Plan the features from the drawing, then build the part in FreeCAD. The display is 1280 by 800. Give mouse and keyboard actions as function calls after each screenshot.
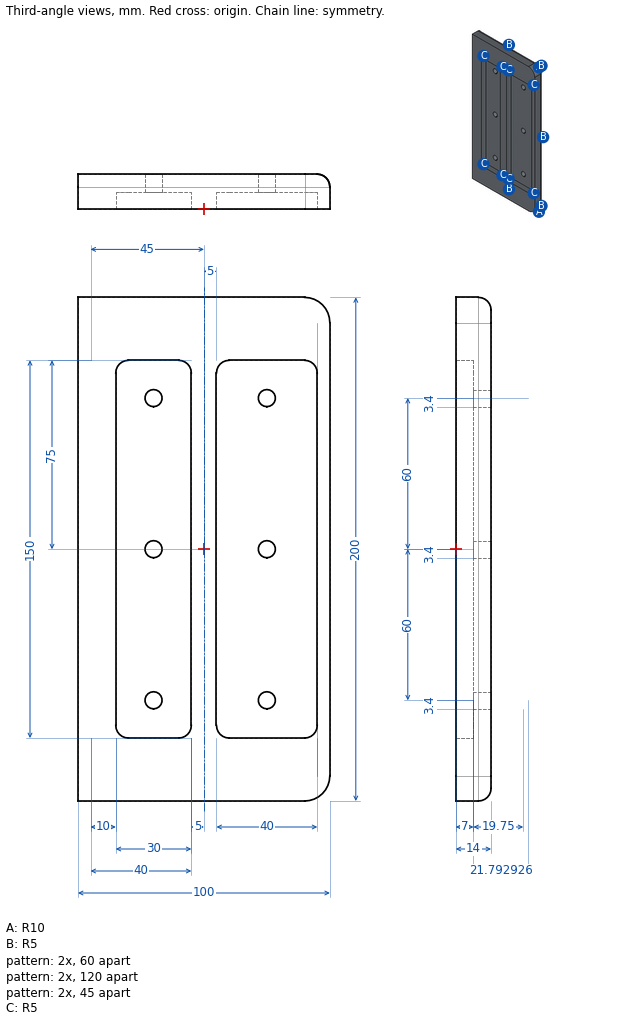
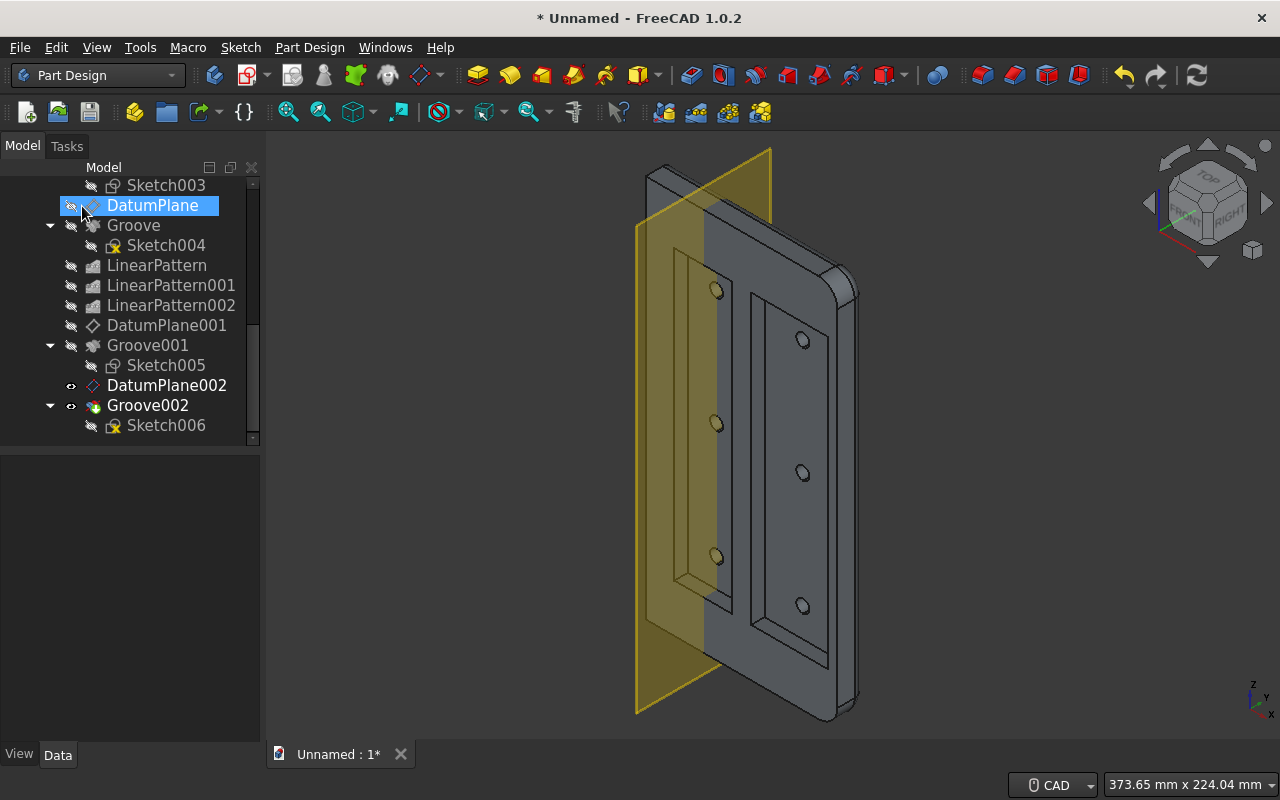
click(116, 386)
key(space)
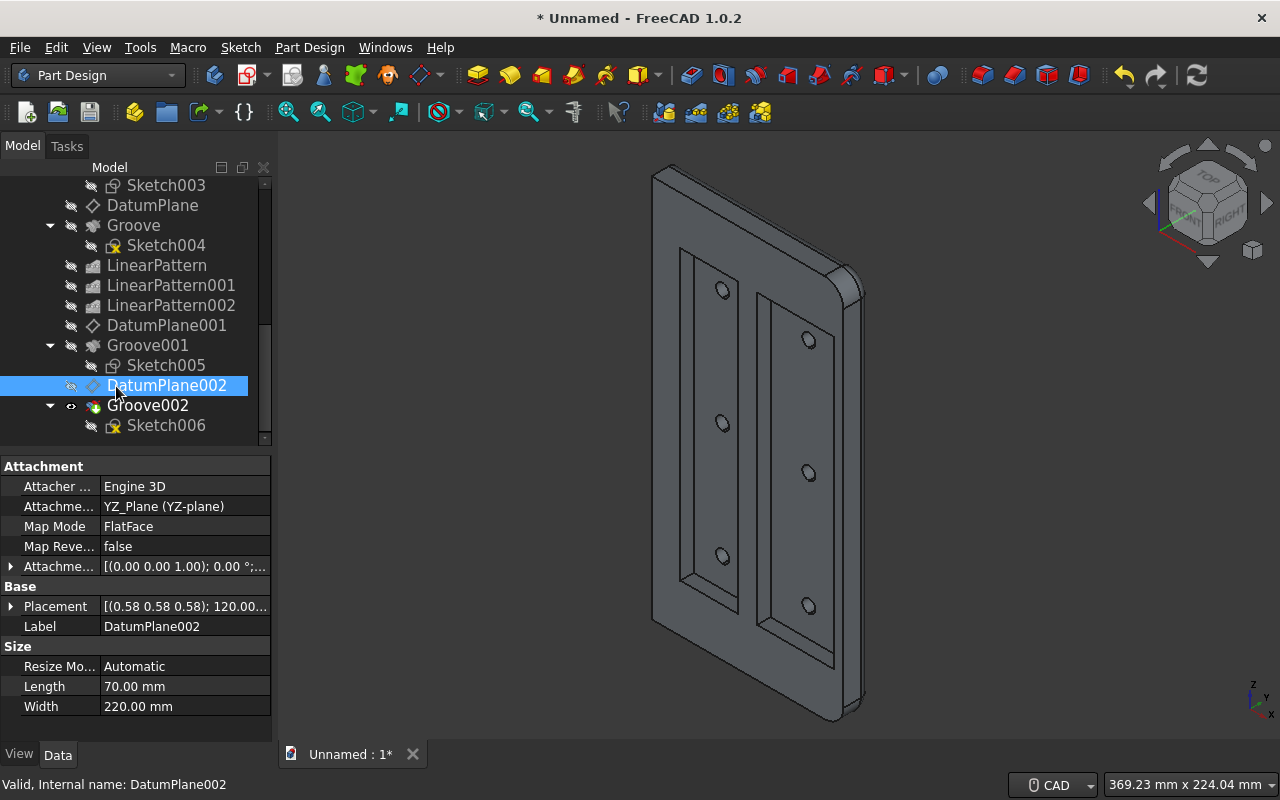
scroll(841, 332, up, 4)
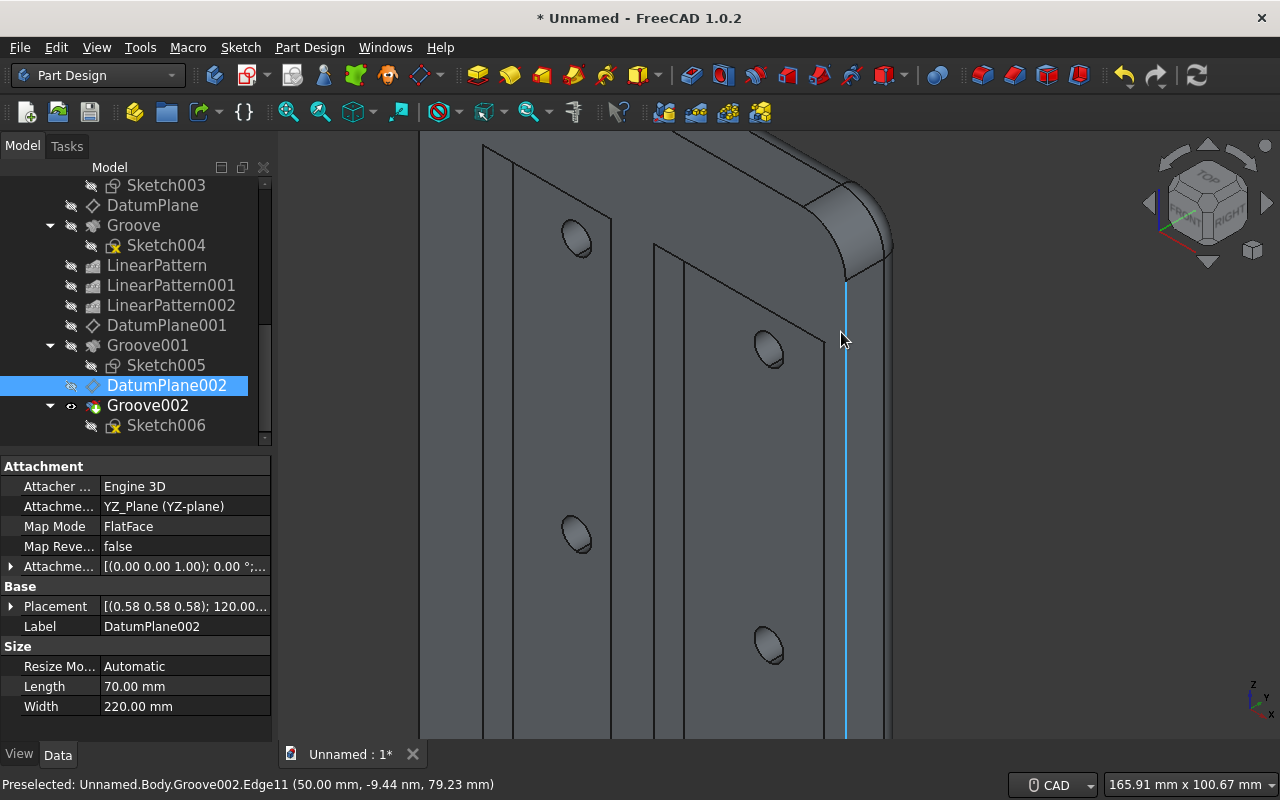
click(290, 112)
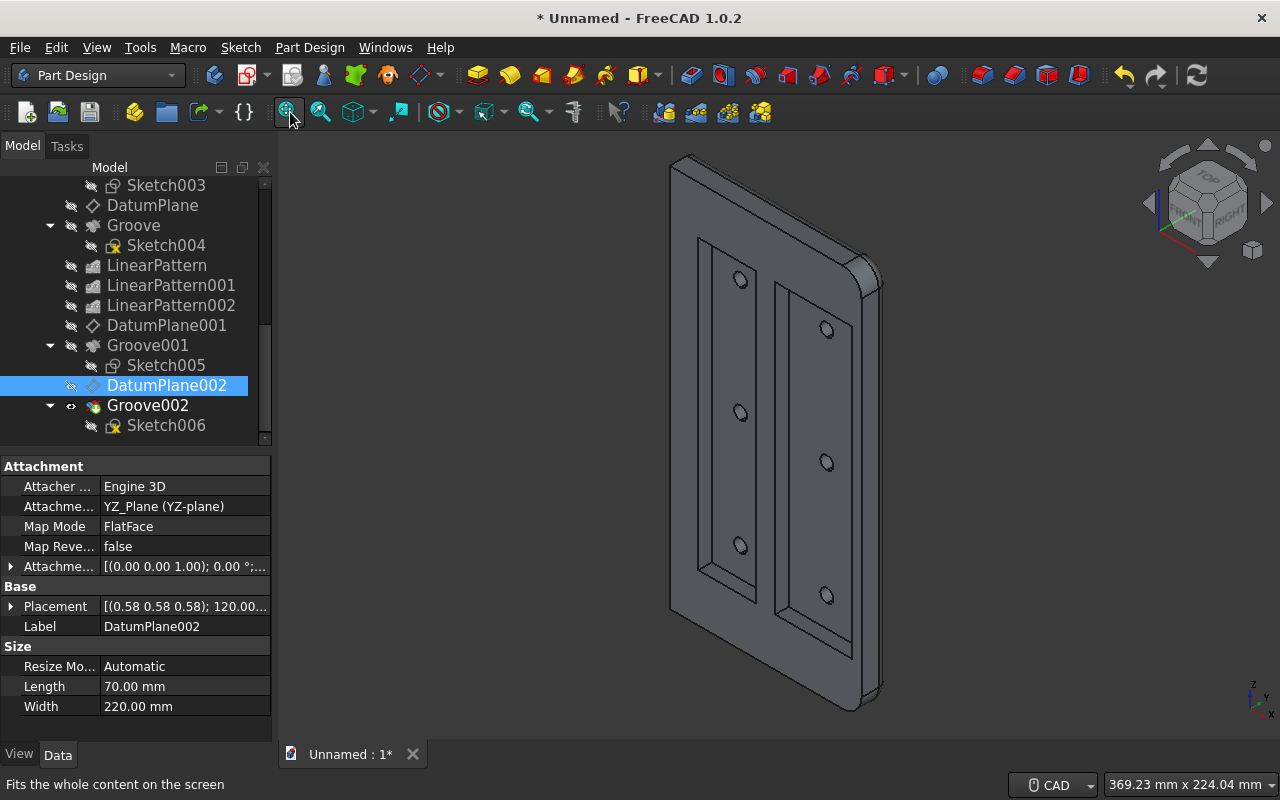
key(2)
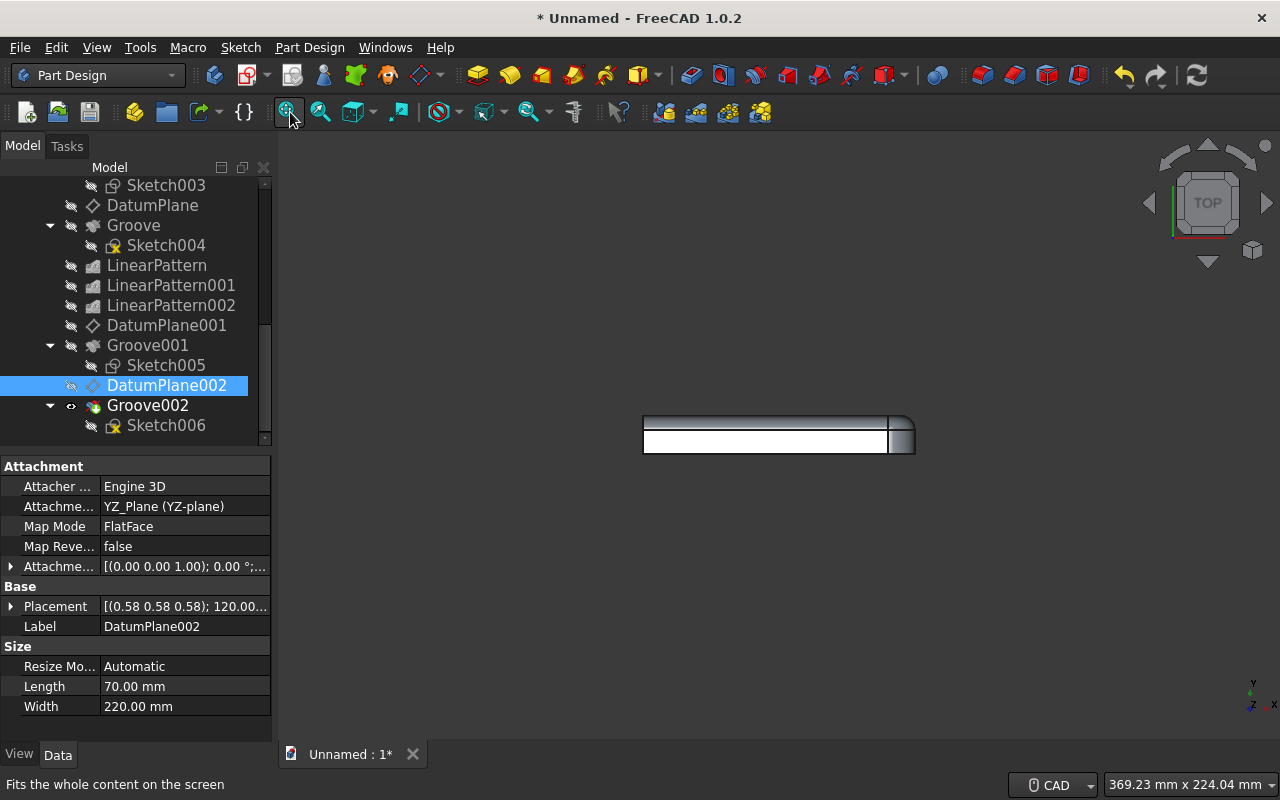
click(290, 112)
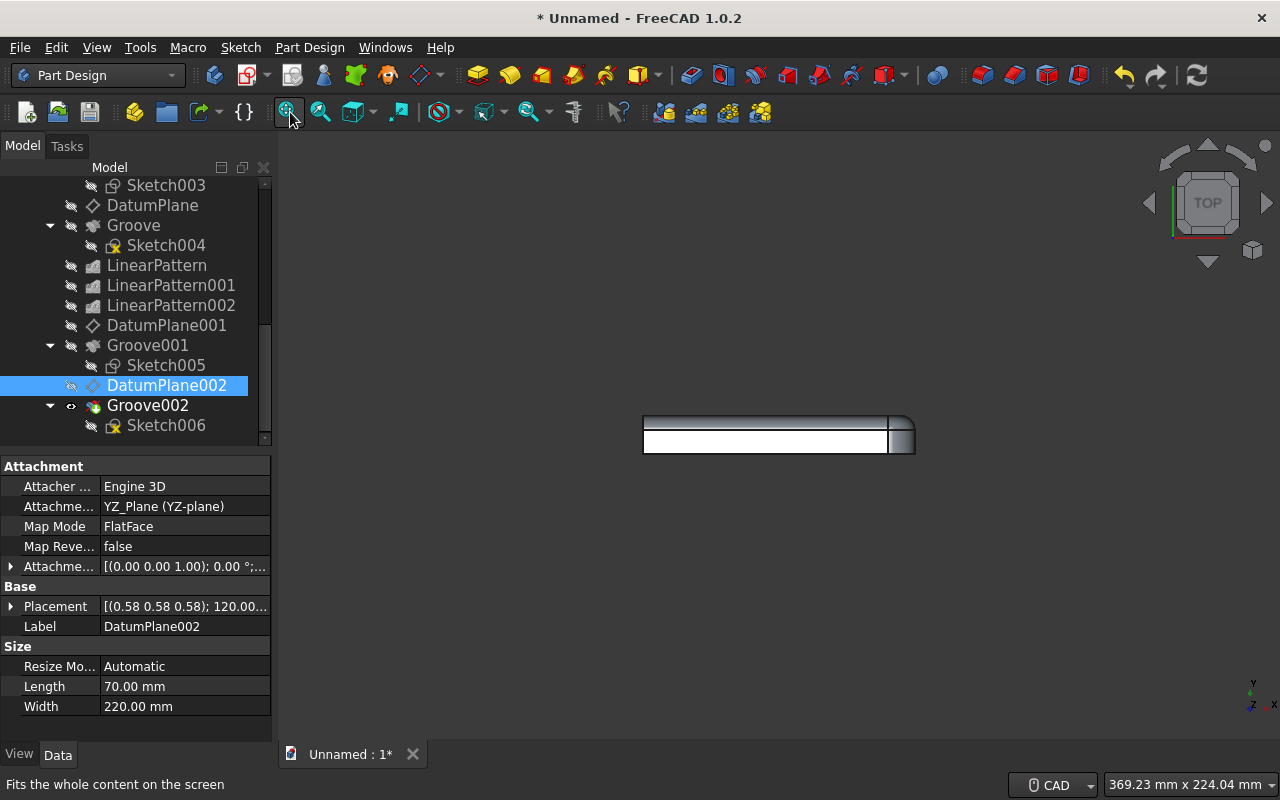
scroll(901, 443, up, 4)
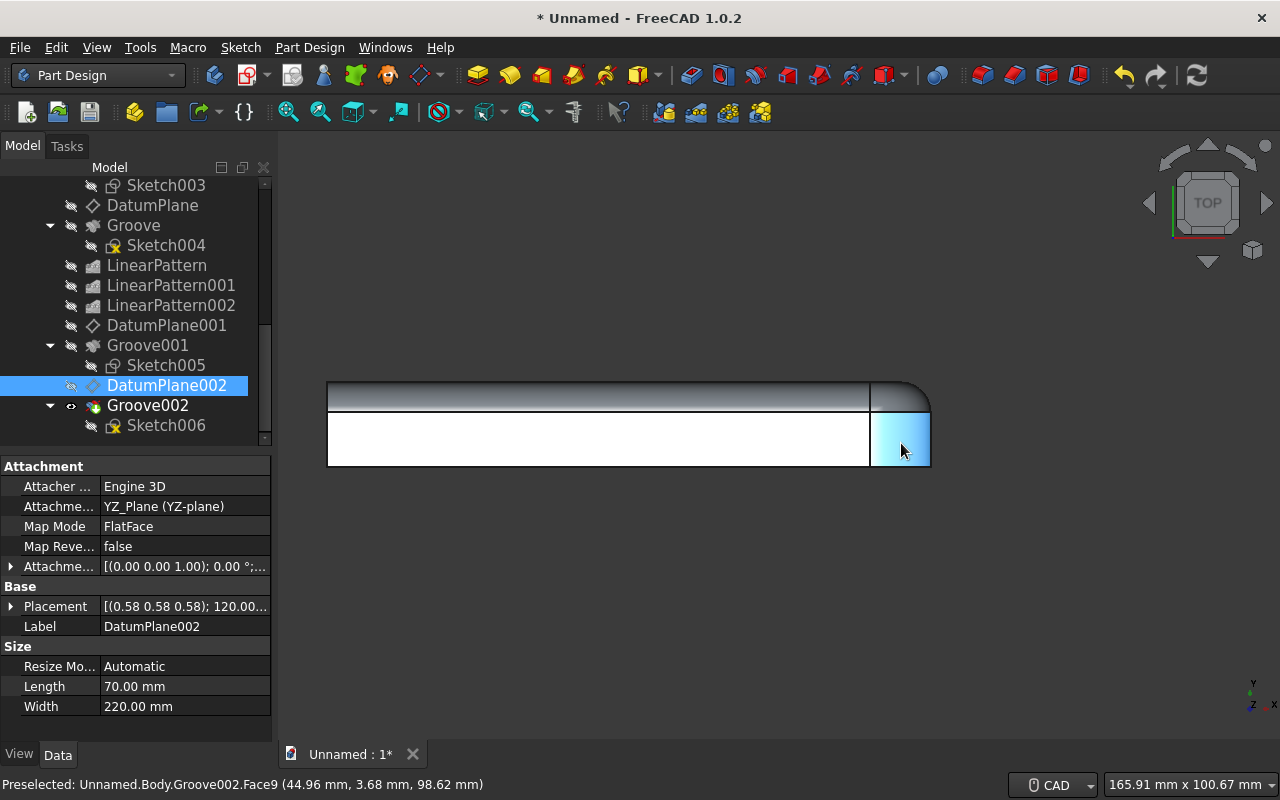
click(290, 112)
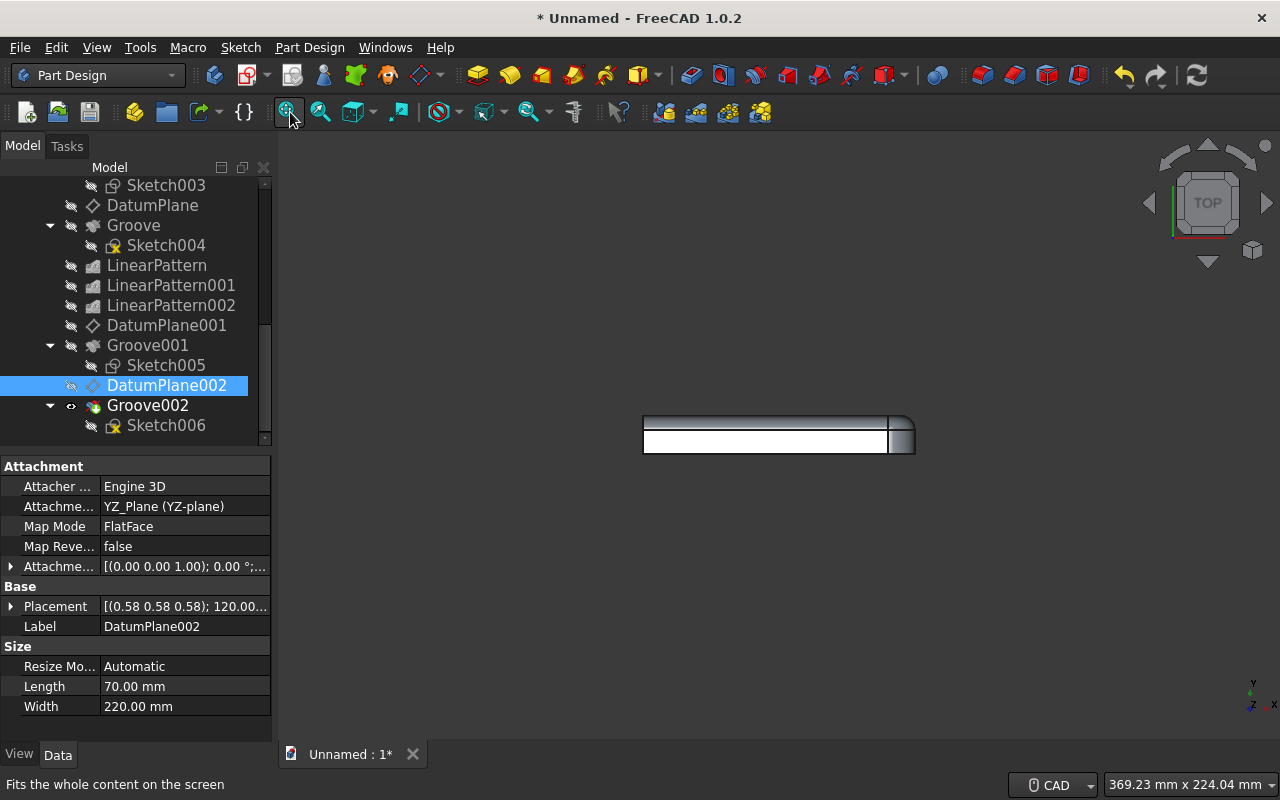
key(0)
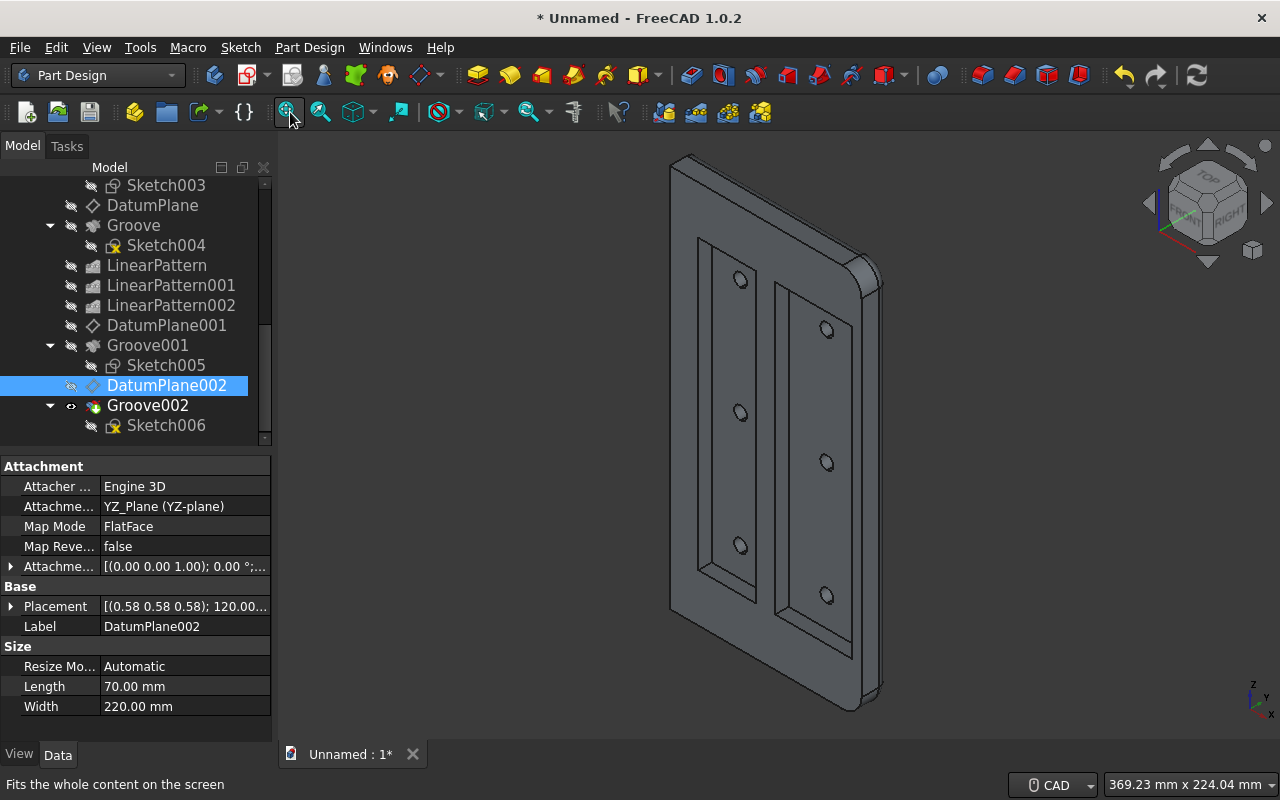
scroll(859, 322, up, 4)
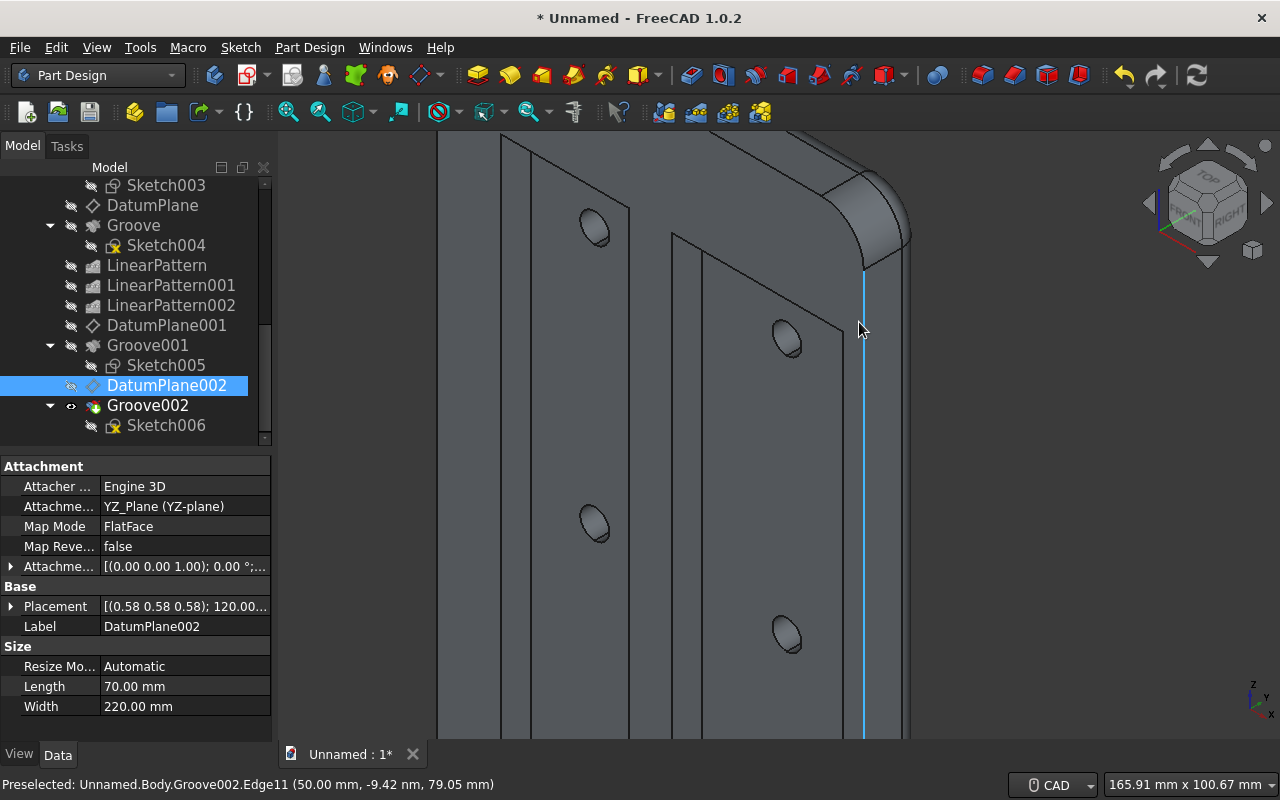
click(290, 112)